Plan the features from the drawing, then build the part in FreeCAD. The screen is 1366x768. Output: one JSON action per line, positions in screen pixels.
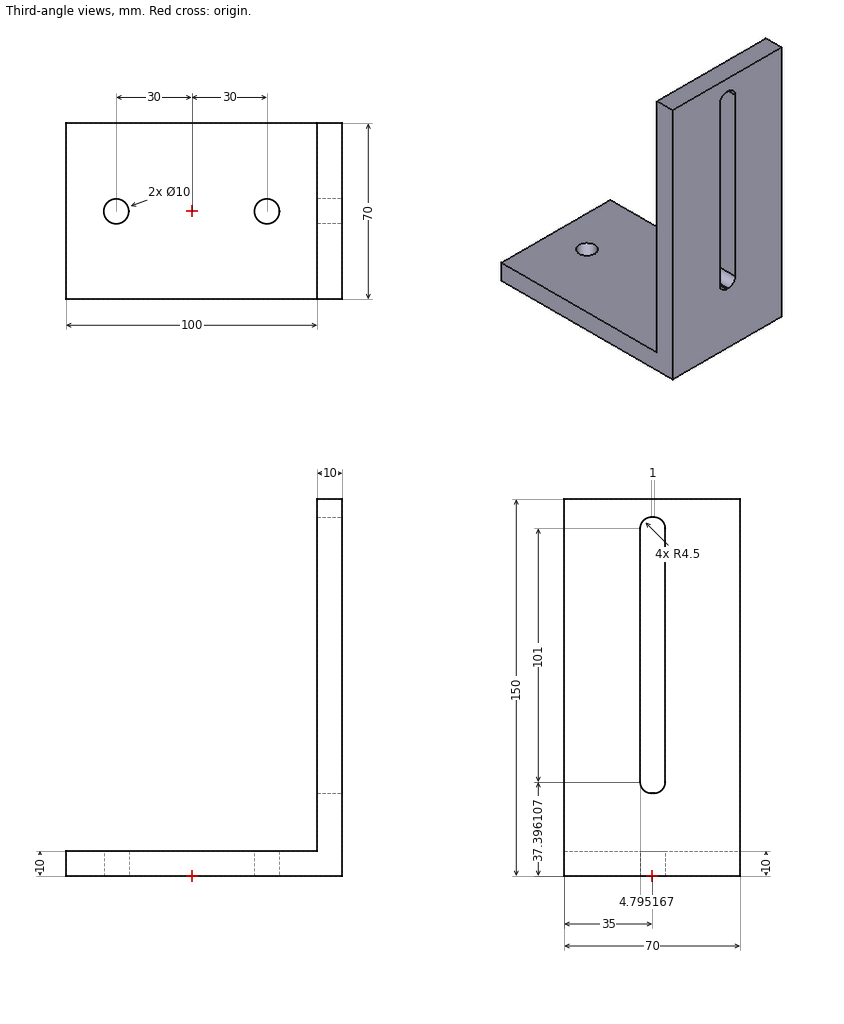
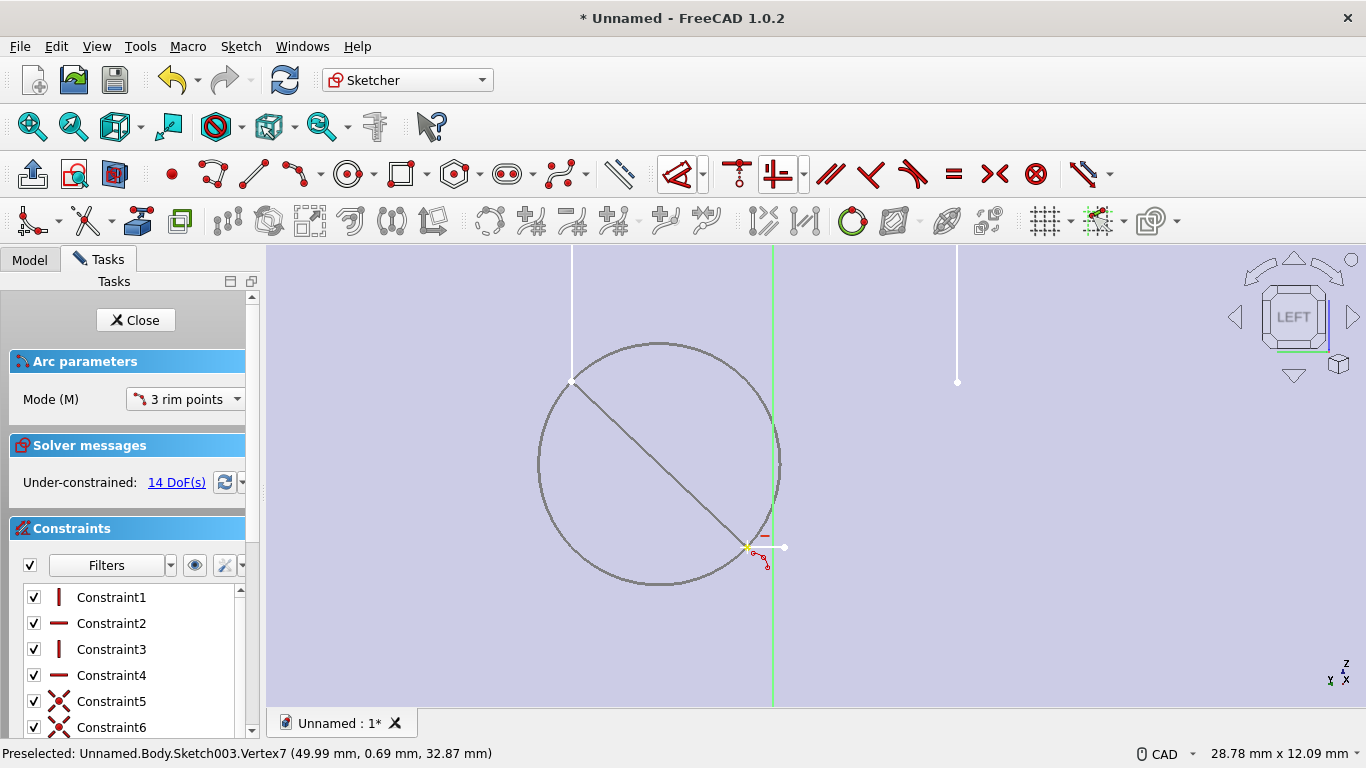
{"action": "scroll", "coordinate": [747, 550], "scroll_direction": "down", "scroll_amount": 15}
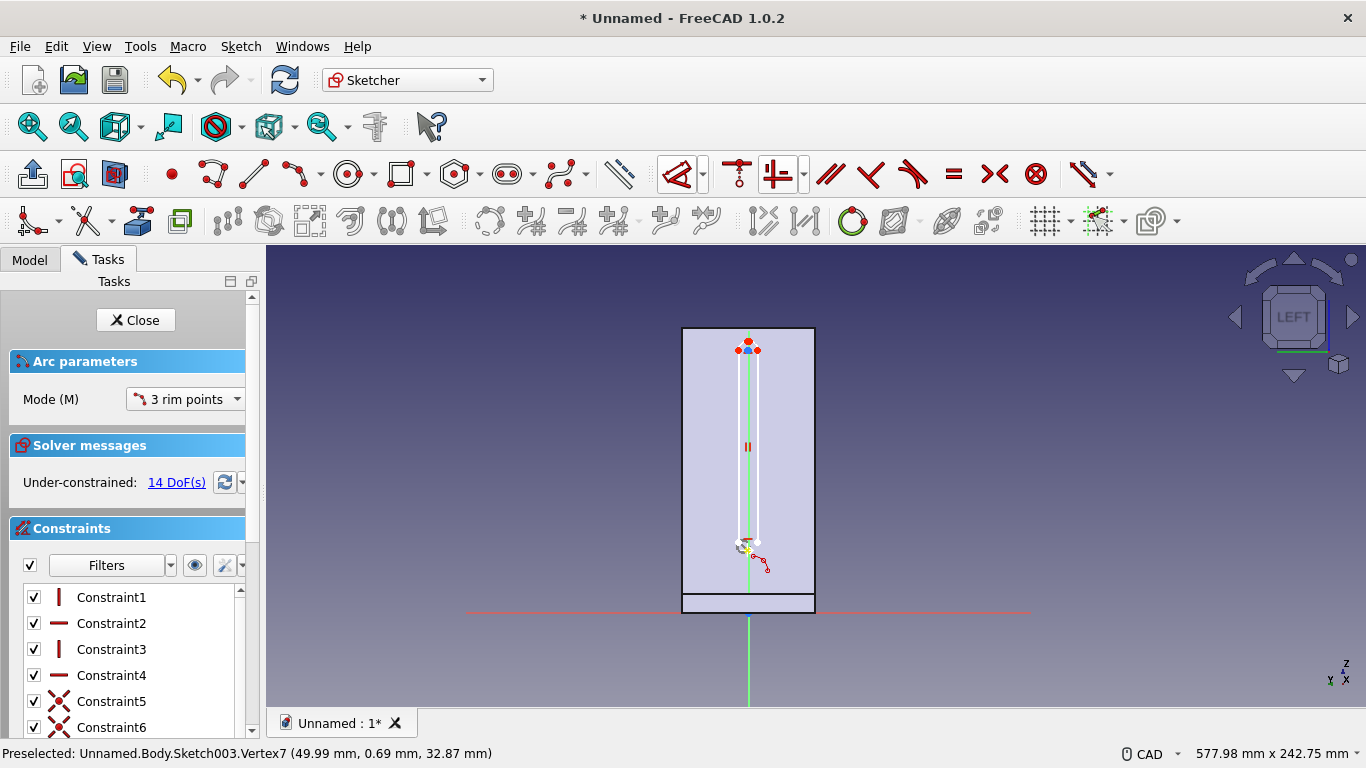
{"action": "scroll", "coordinate": [741, 548], "scroll_direction": "up", "scroll_amount": 10}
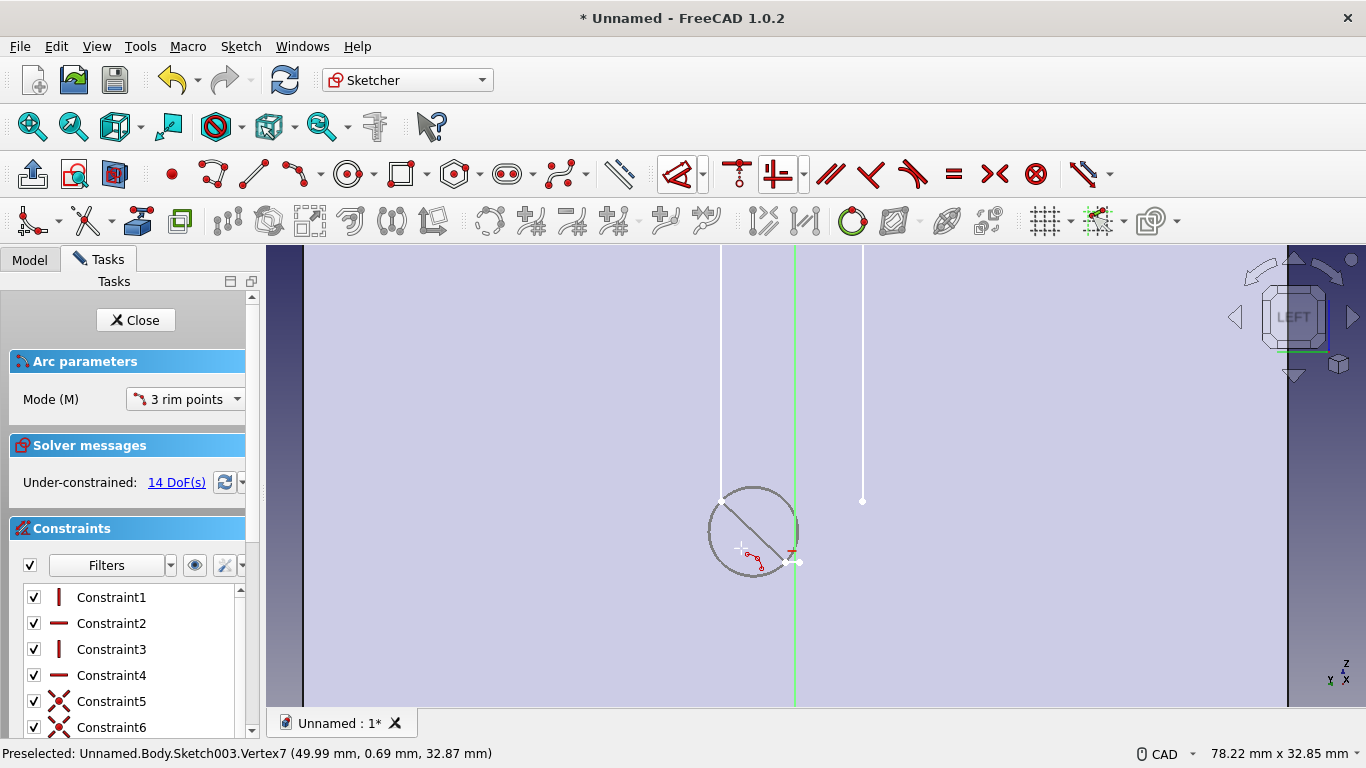
{"action": "left_click", "coordinate": [741, 543]}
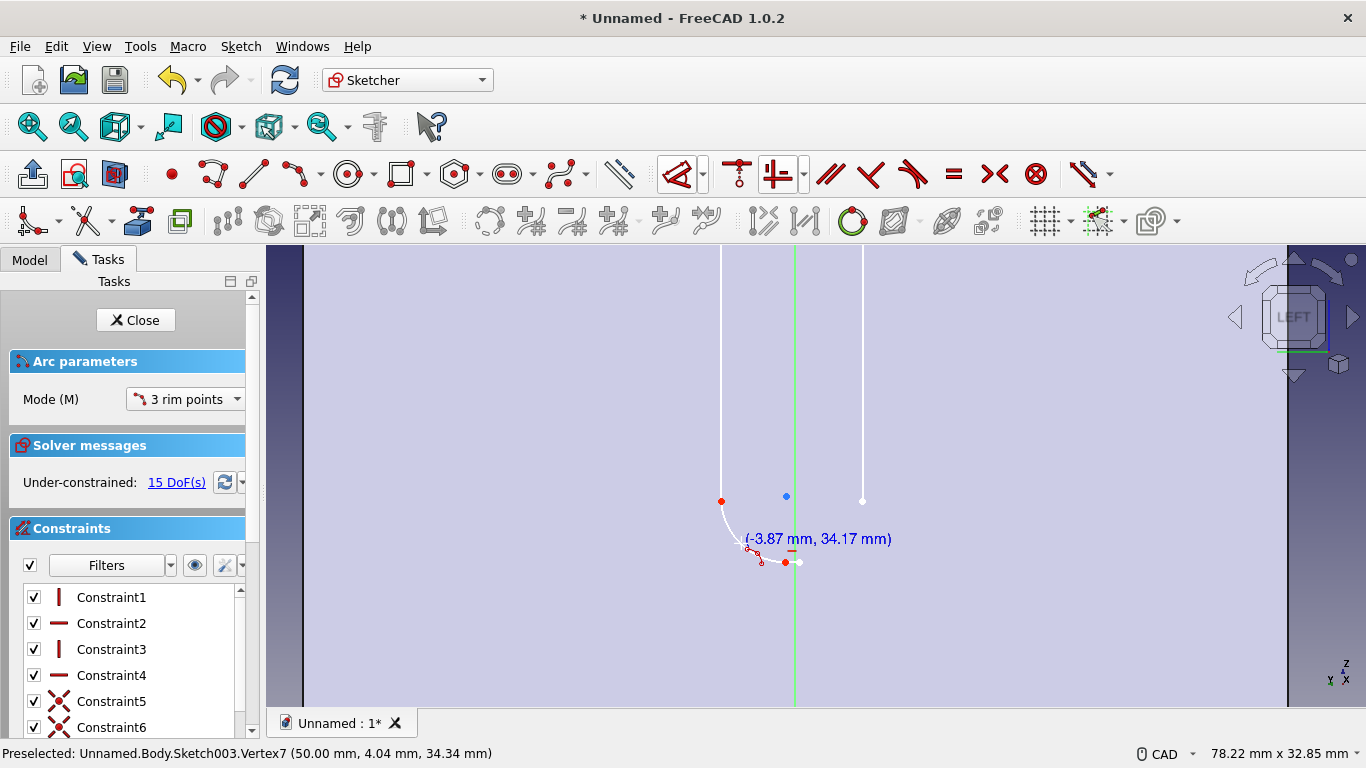
{"action": "scroll", "coordinate": [800, 562], "scroll_direction": "up", "scroll_amount": 7}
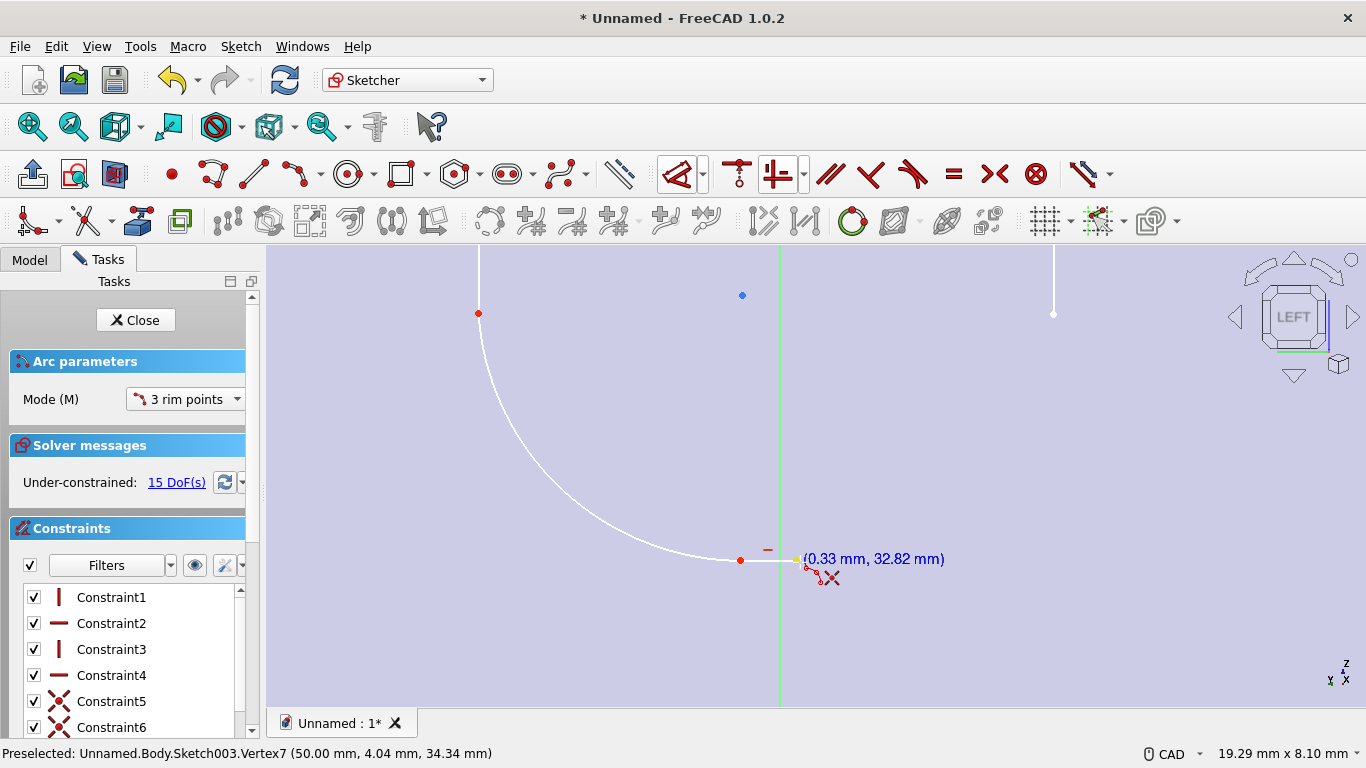
{"action": "left_click", "coordinate": [797, 561]}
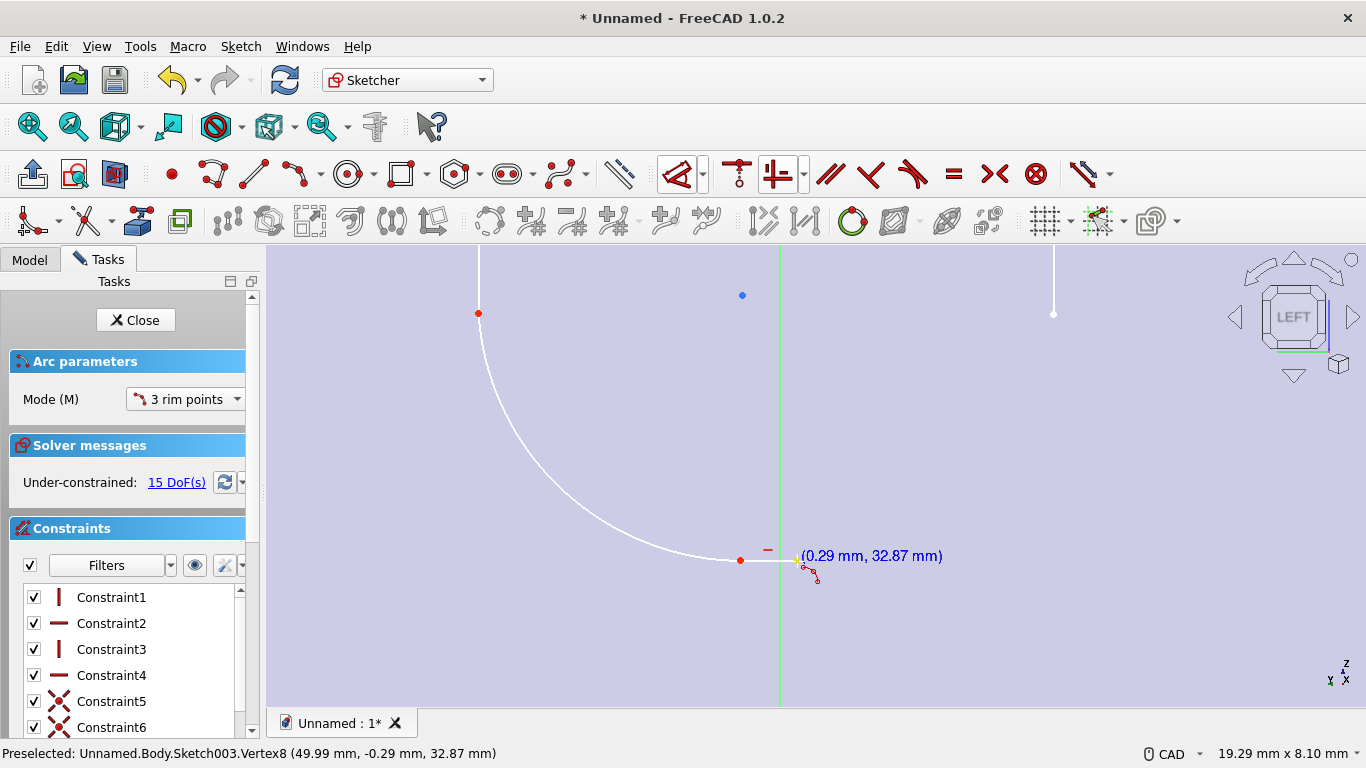
{"action": "scroll", "coordinate": [747, 566], "scroll_direction": "down", "scroll_amount": 16}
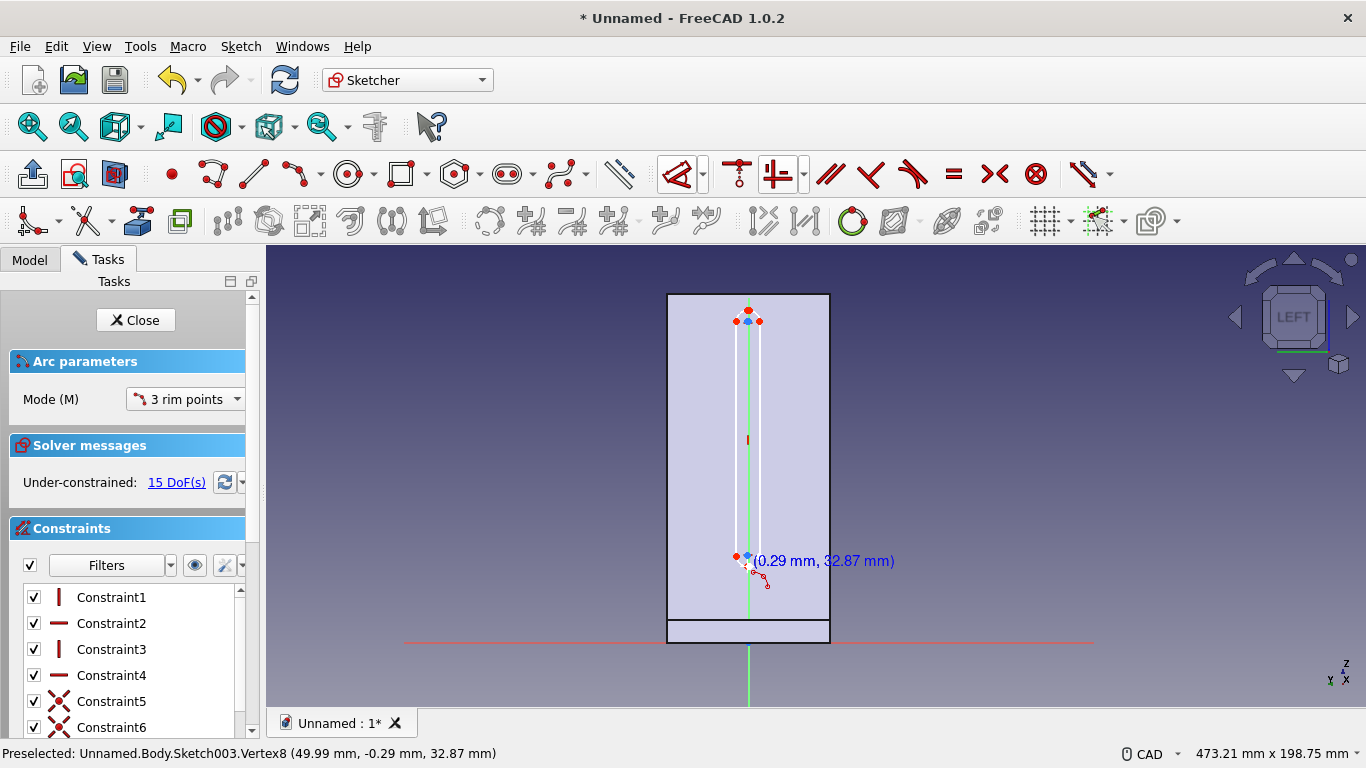
{"action": "scroll", "coordinate": [760, 556], "scroll_direction": "up", "scroll_amount": 2}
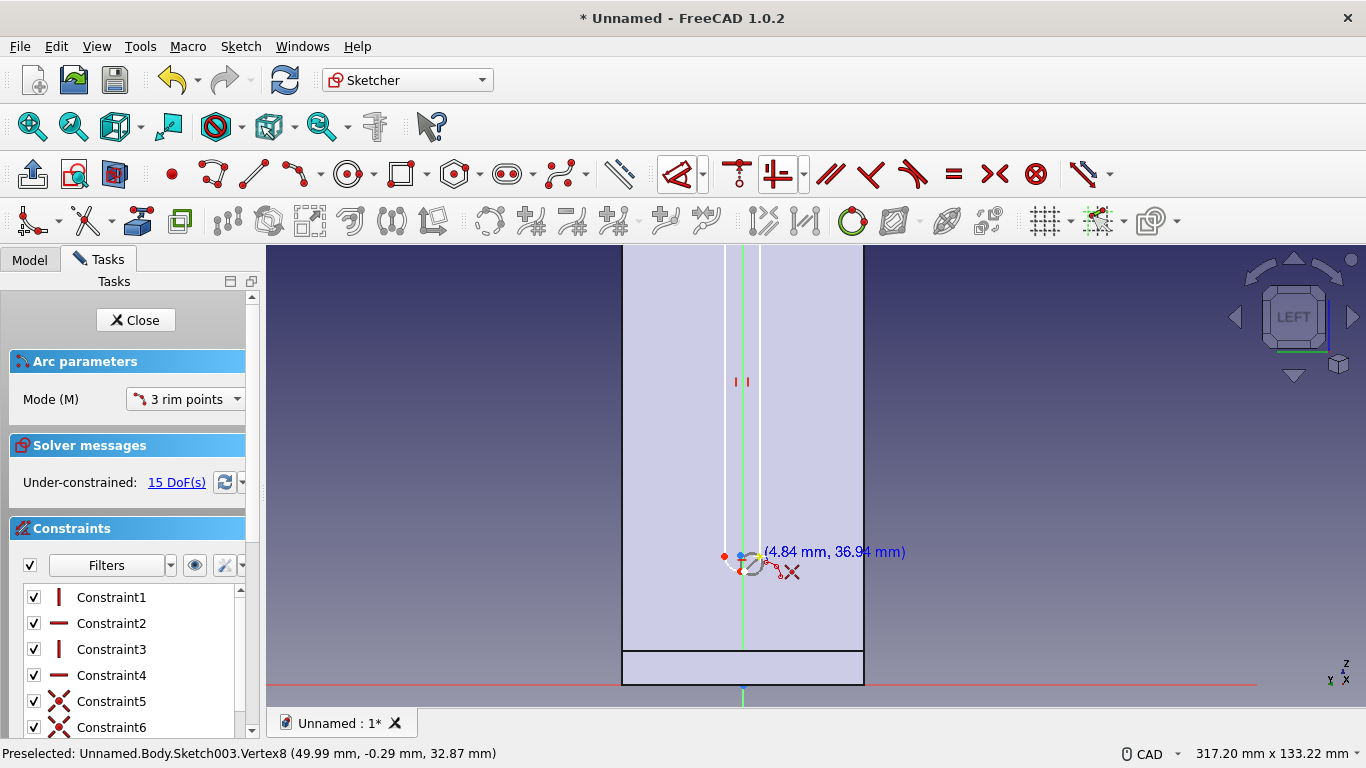
{"action": "left_click", "coordinate": [760, 556]}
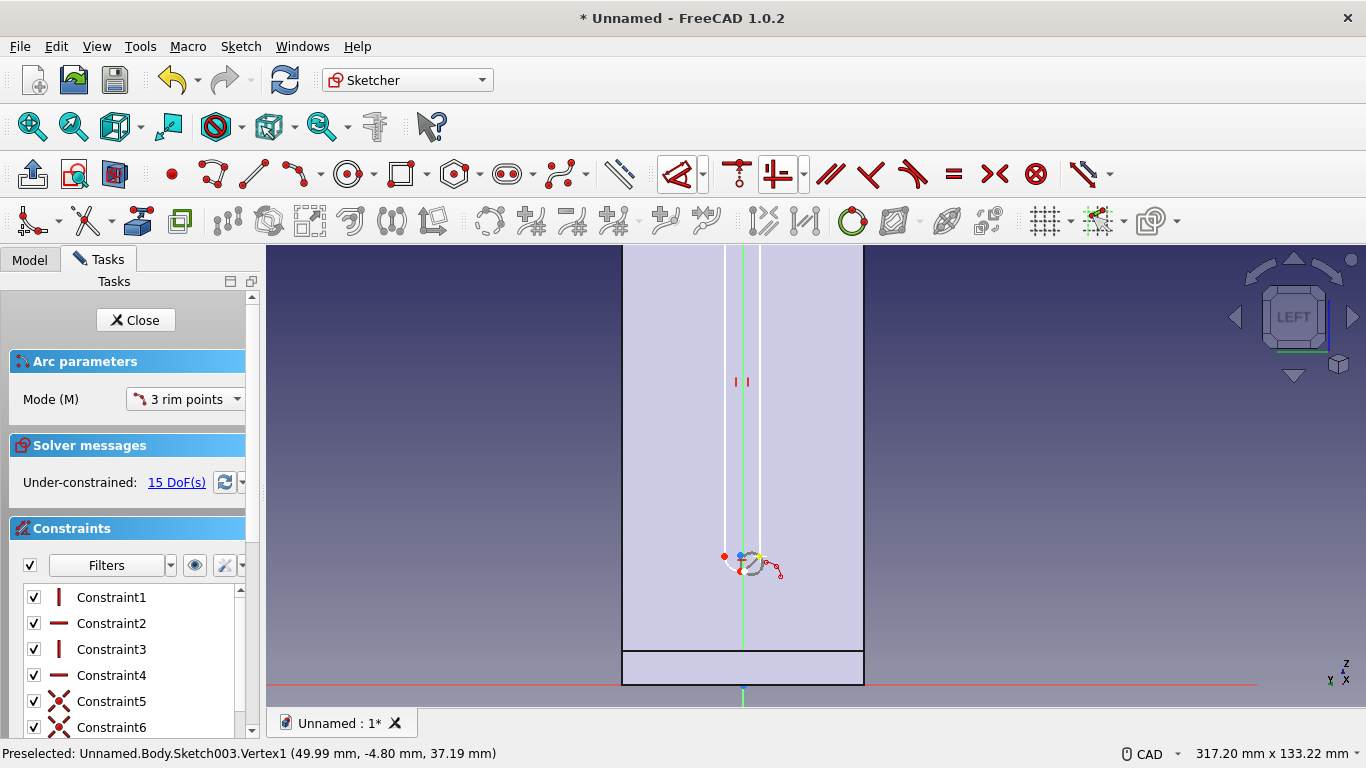
{"action": "scroll", "coordinate": [755, 567], "scroll_direction": "up", "scroll_amount": 7}